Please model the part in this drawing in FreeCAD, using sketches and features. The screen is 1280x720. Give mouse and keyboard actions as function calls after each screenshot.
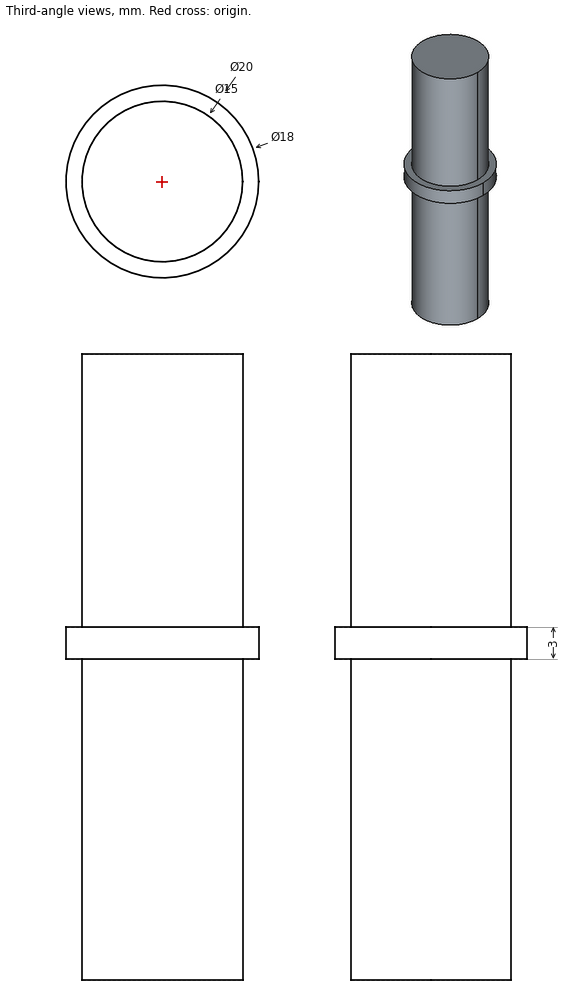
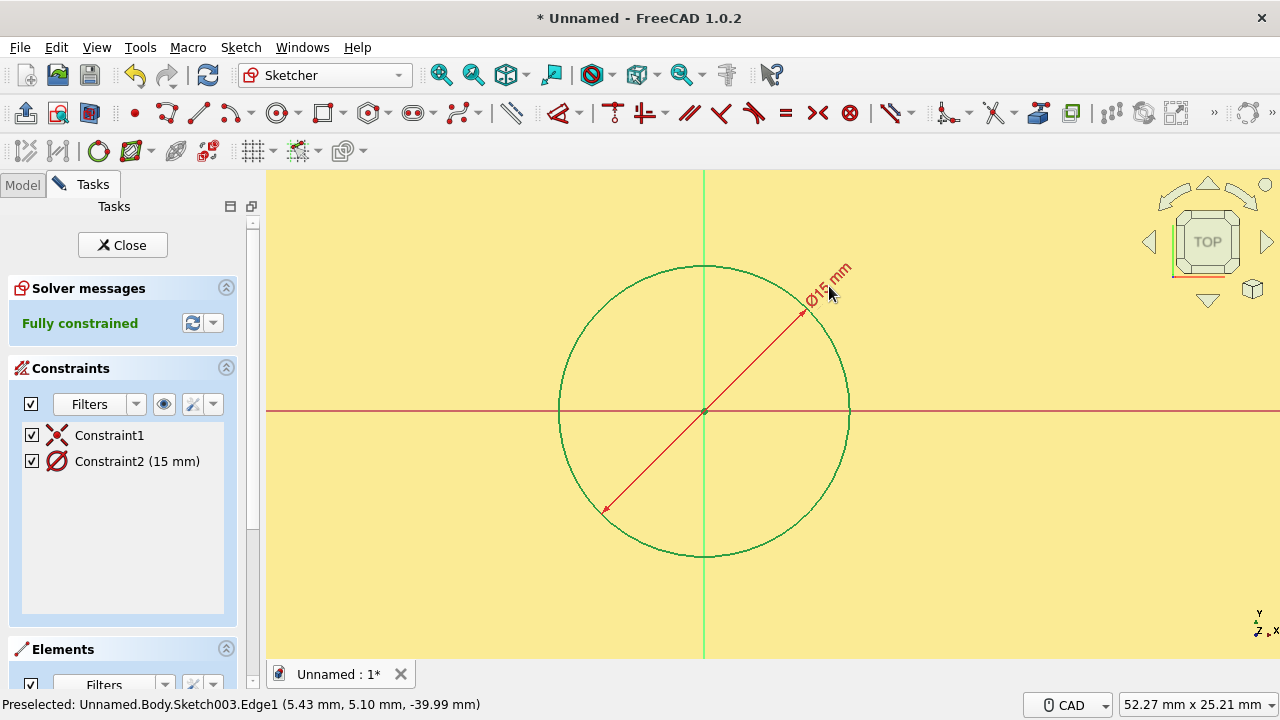
click(123, 245)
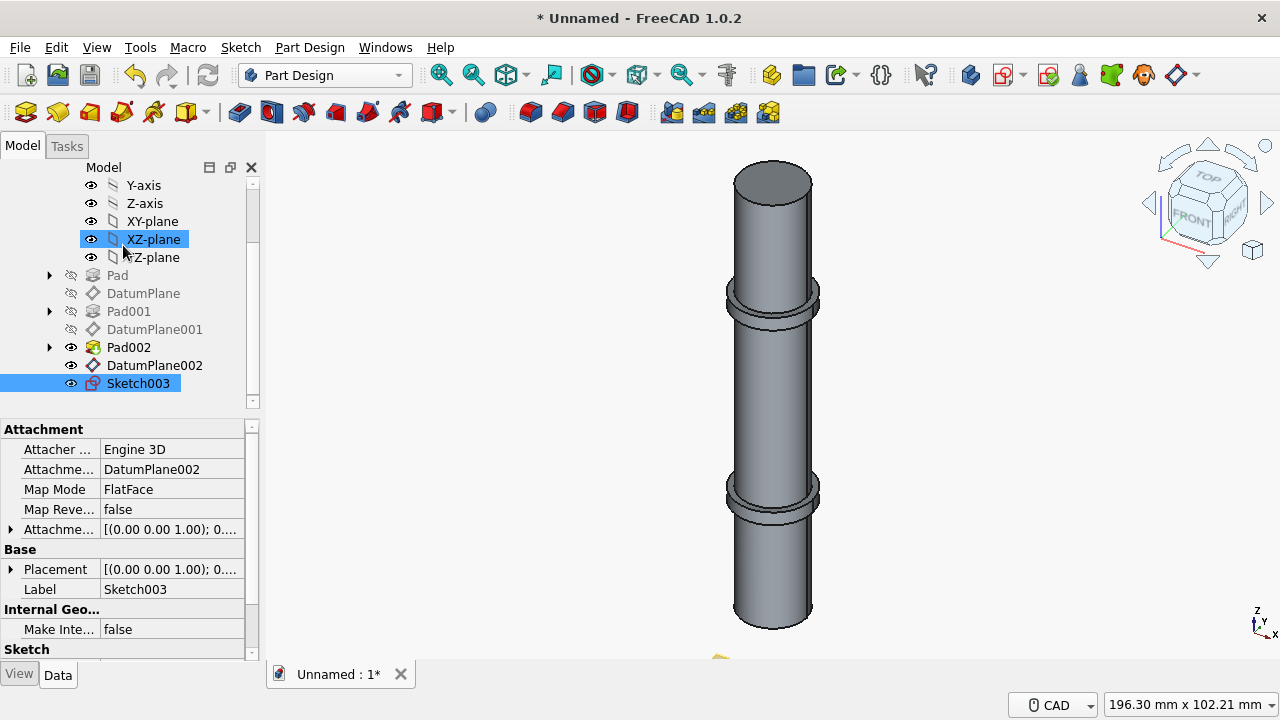
click(26, 112)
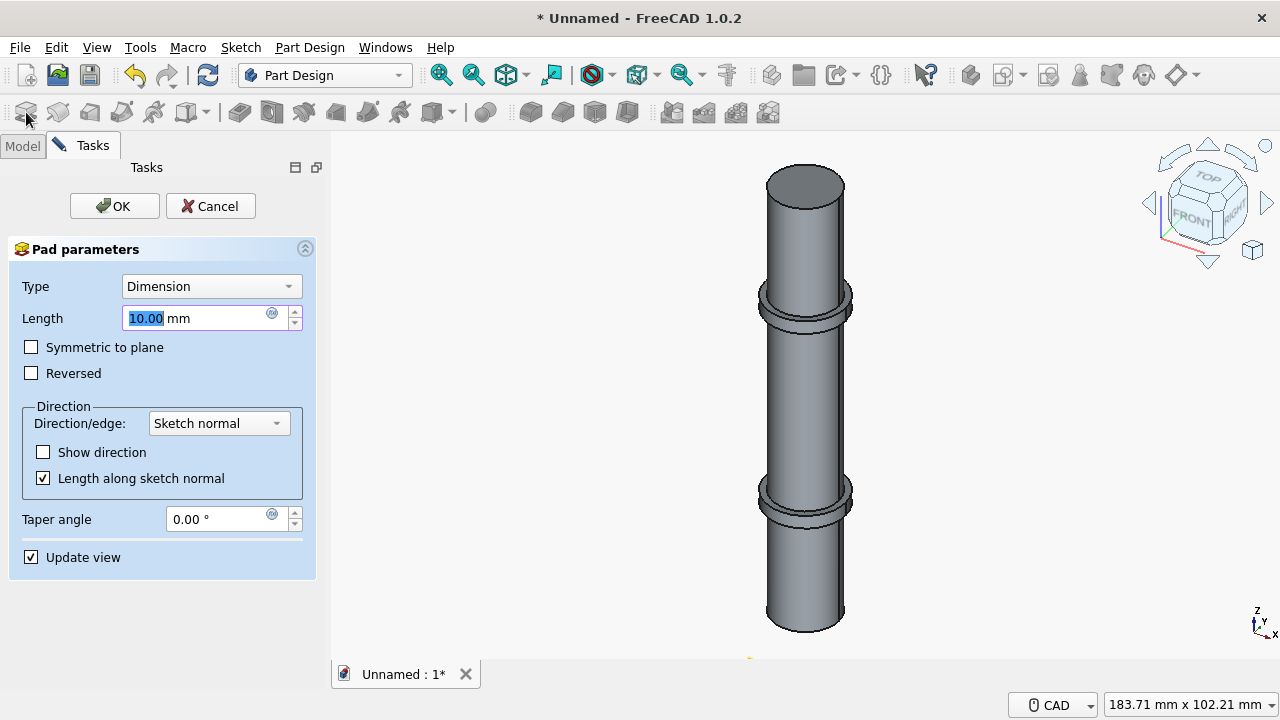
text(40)
key(Tab)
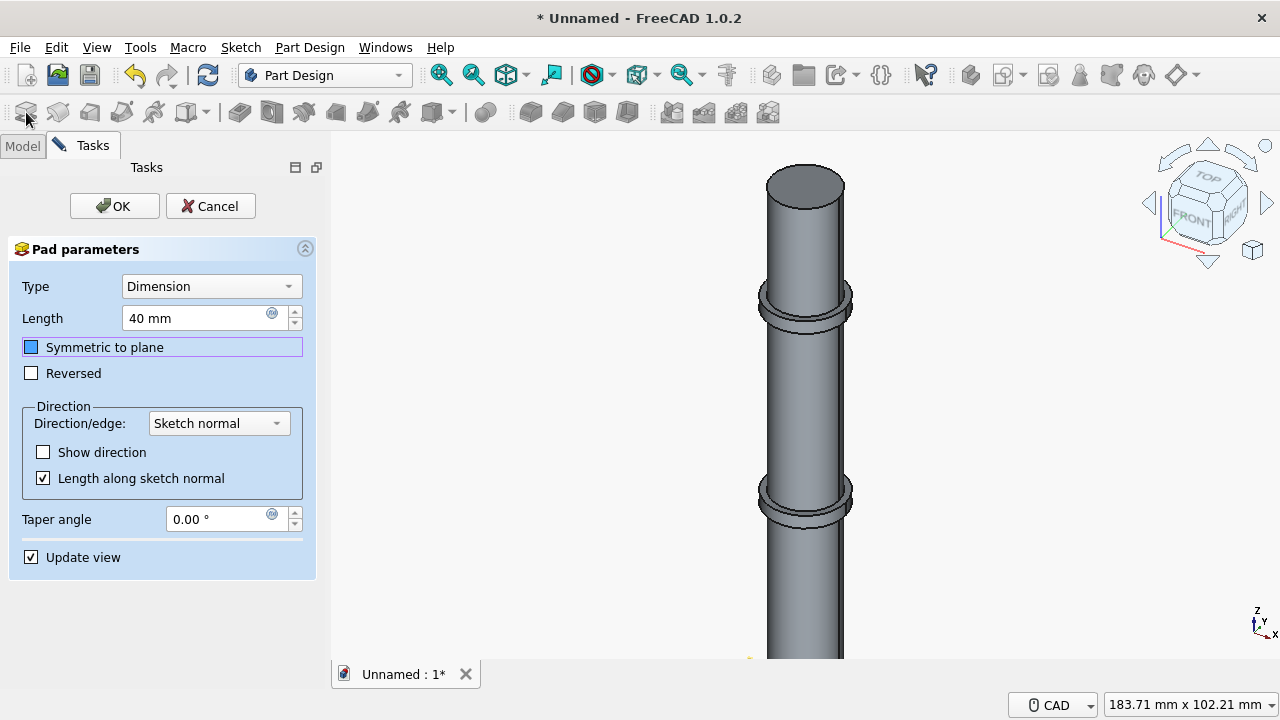
click(115, 206)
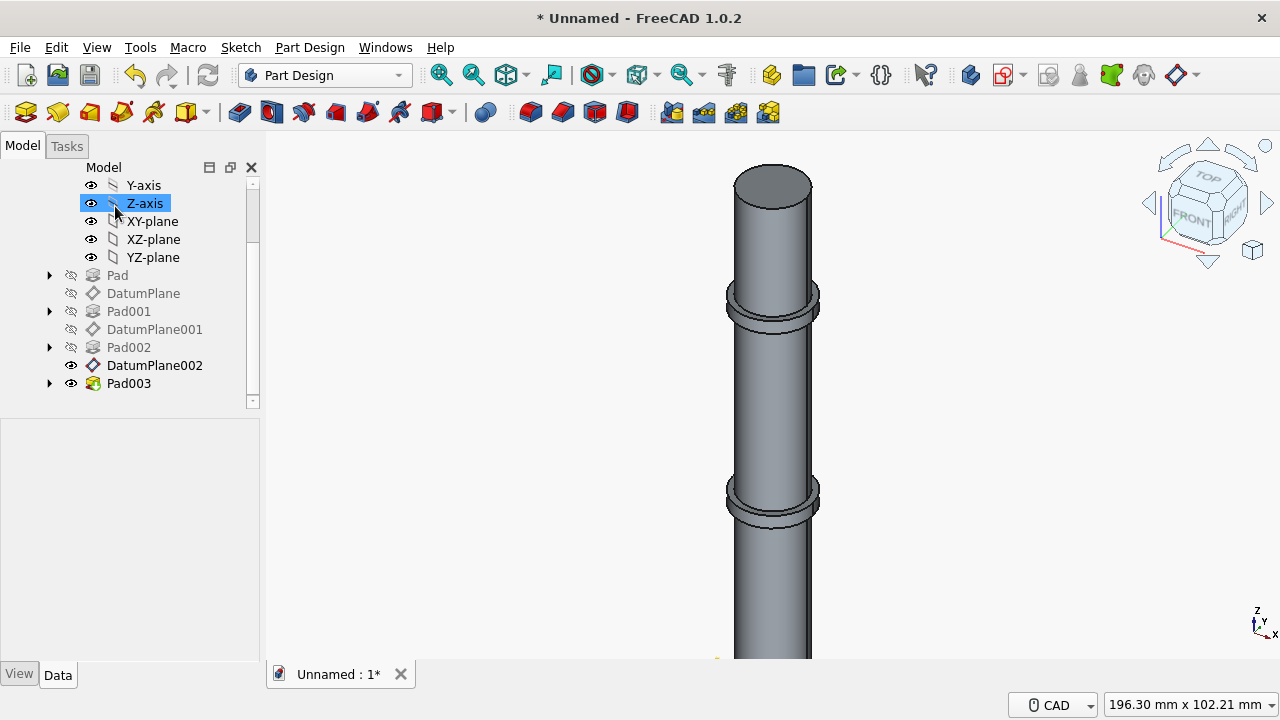
click(116, 365)
key(space)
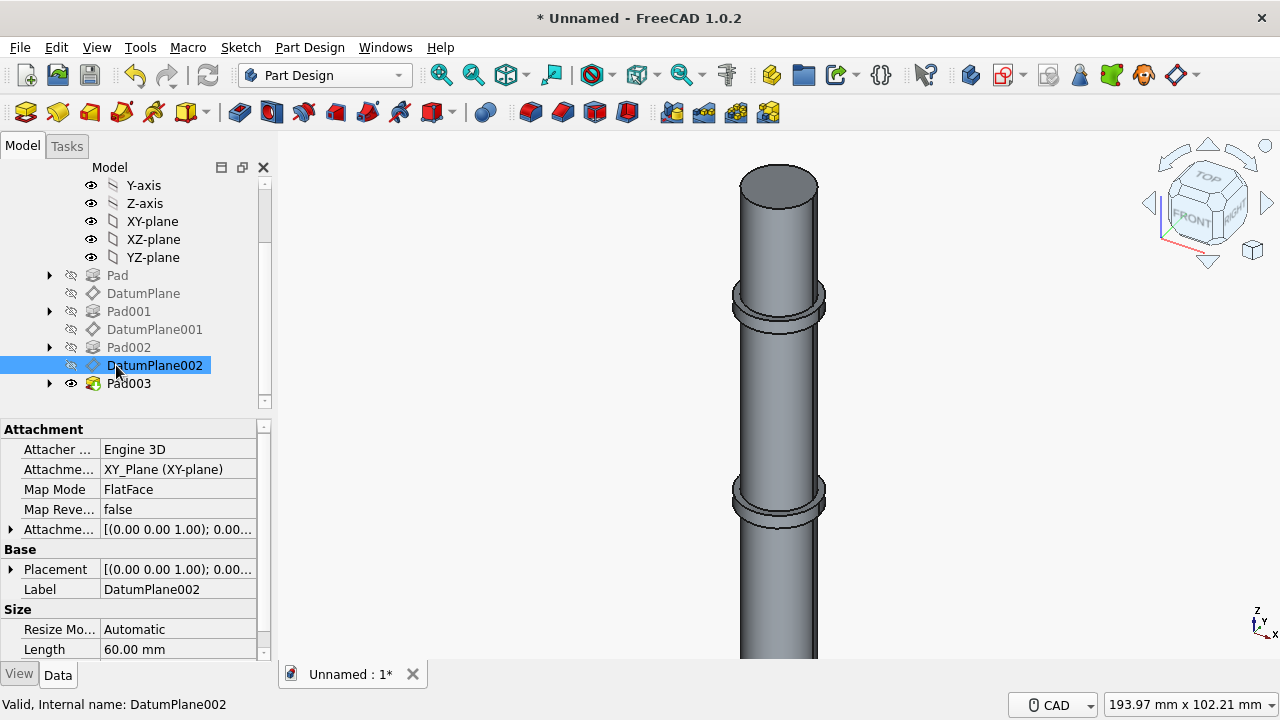
key(v)
key(f)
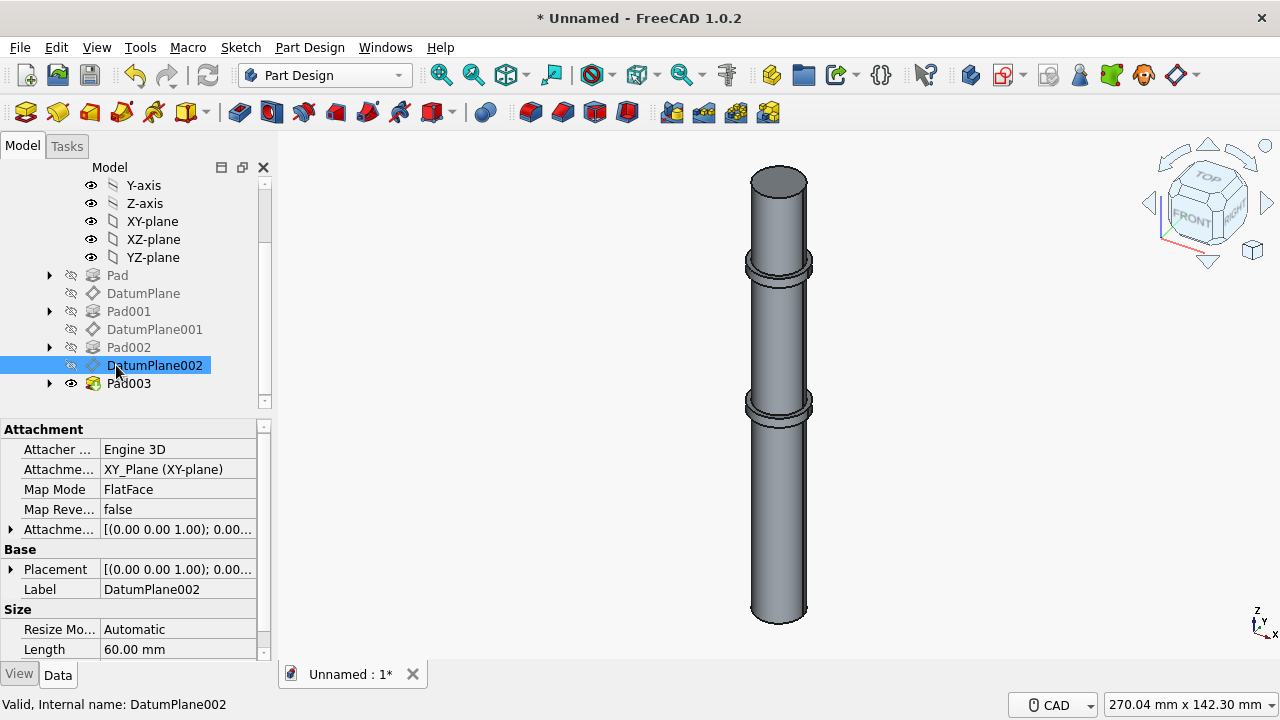
key(5)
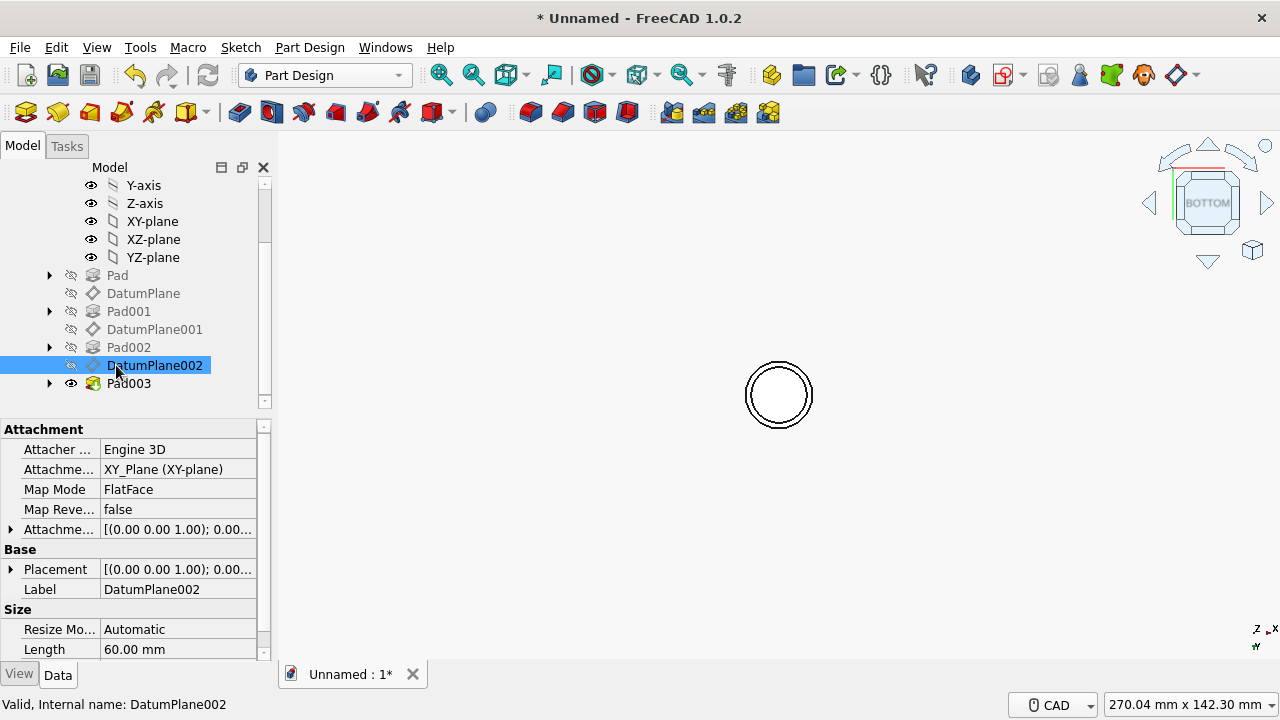
click(442, 76)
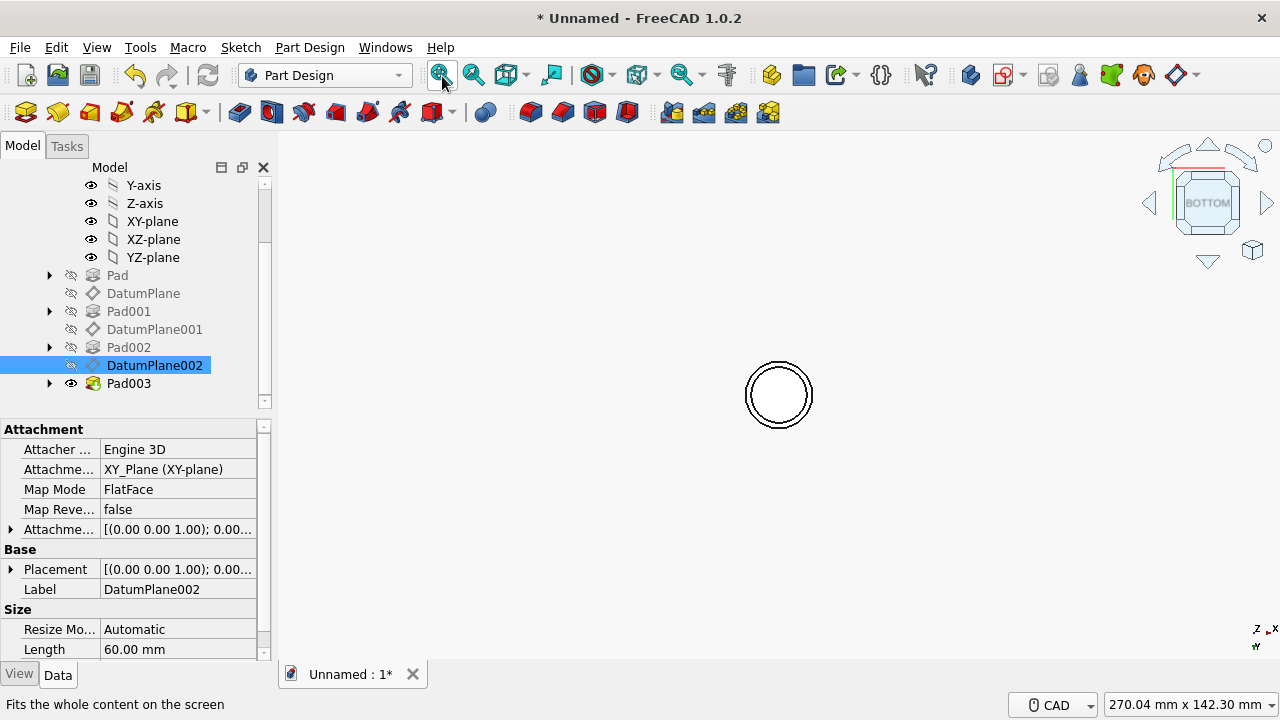
click(779, 394)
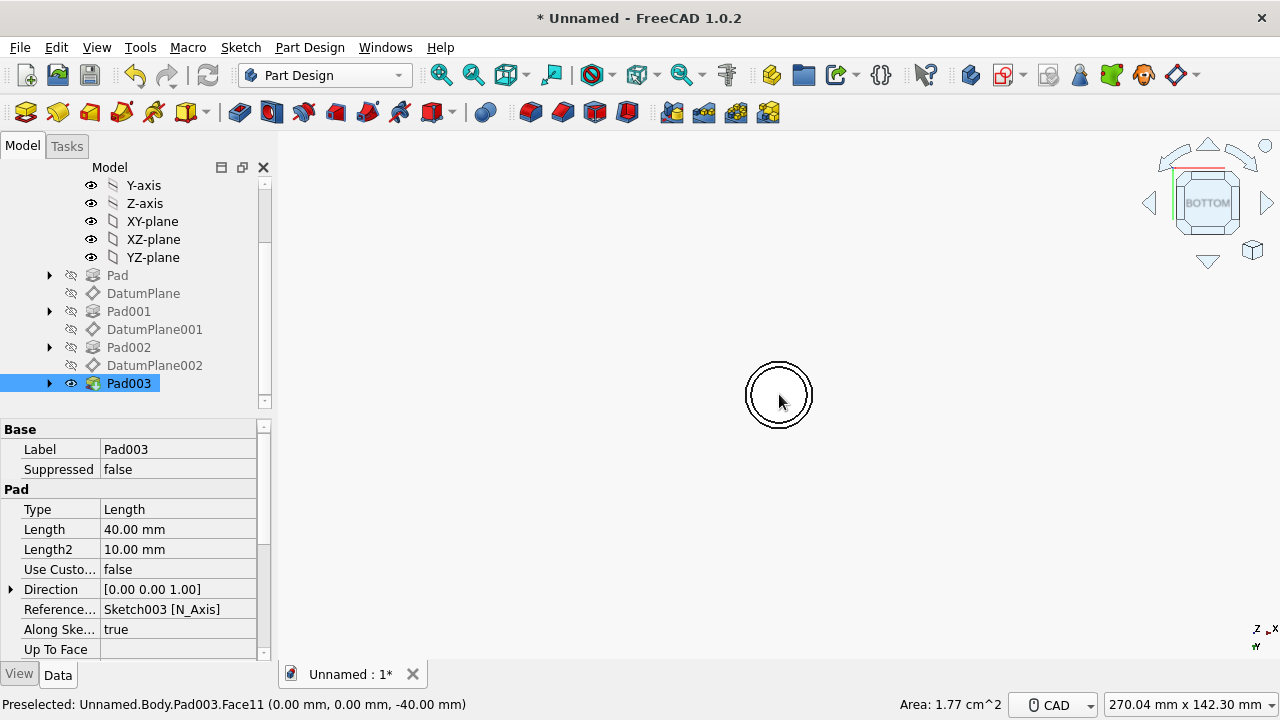
click(1004, 76)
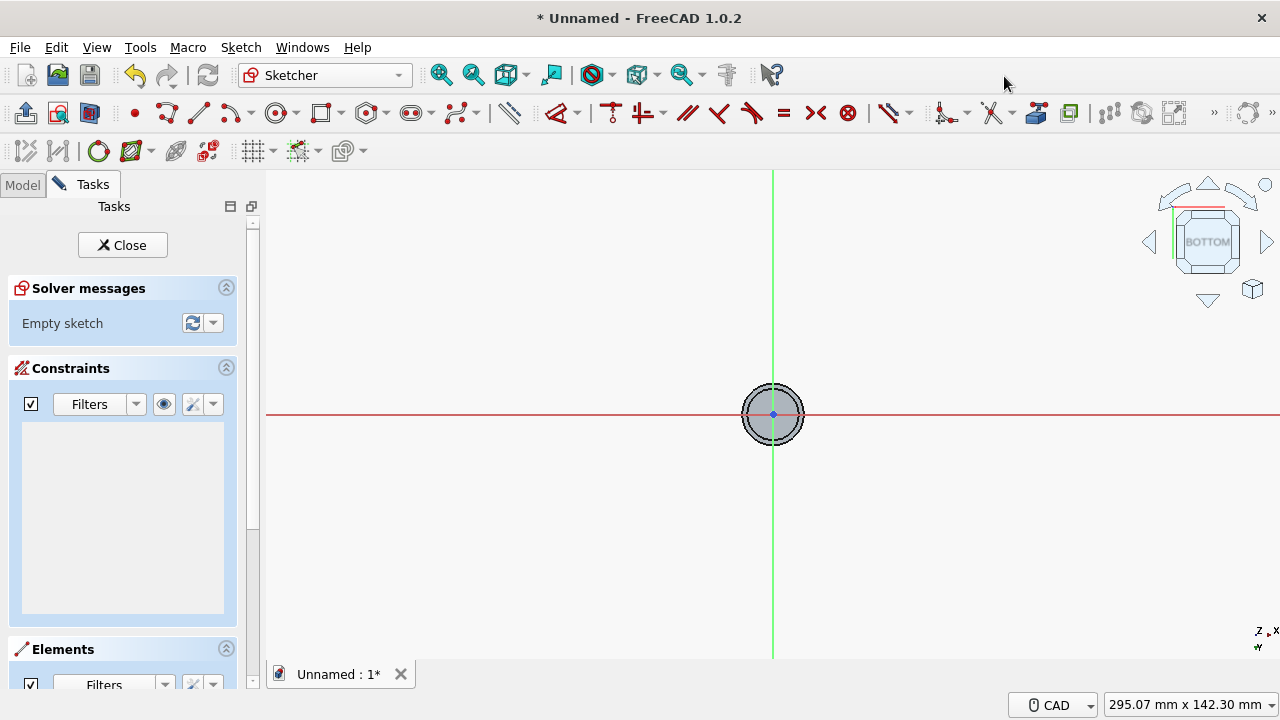
scroll(795, 415, up, 7)